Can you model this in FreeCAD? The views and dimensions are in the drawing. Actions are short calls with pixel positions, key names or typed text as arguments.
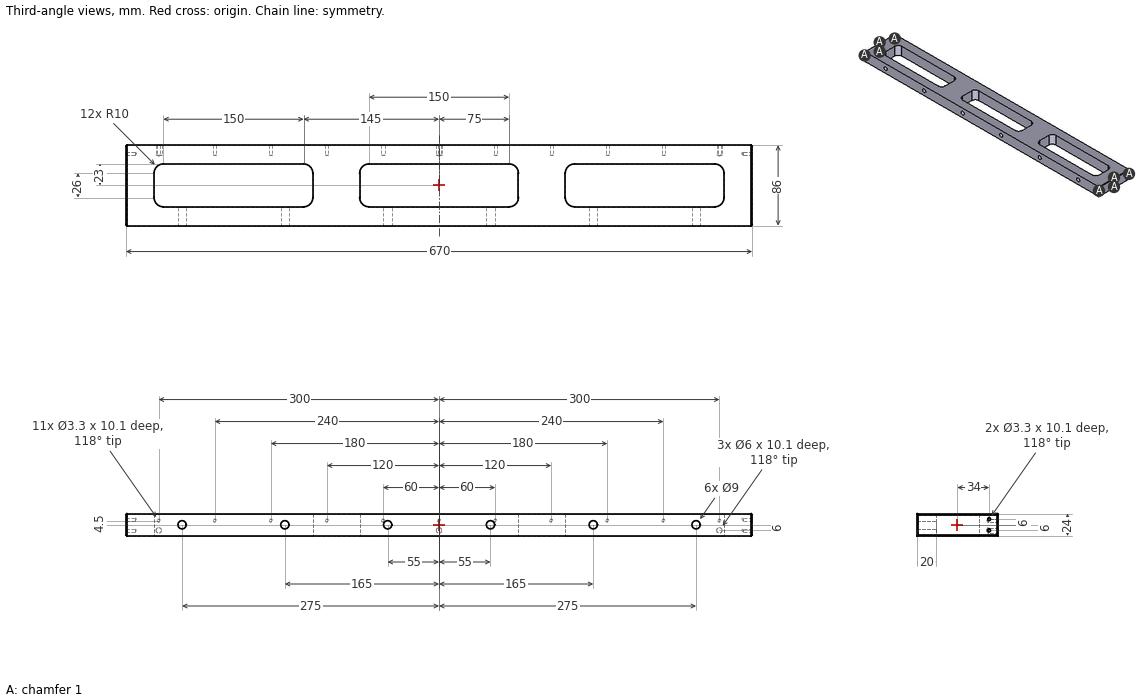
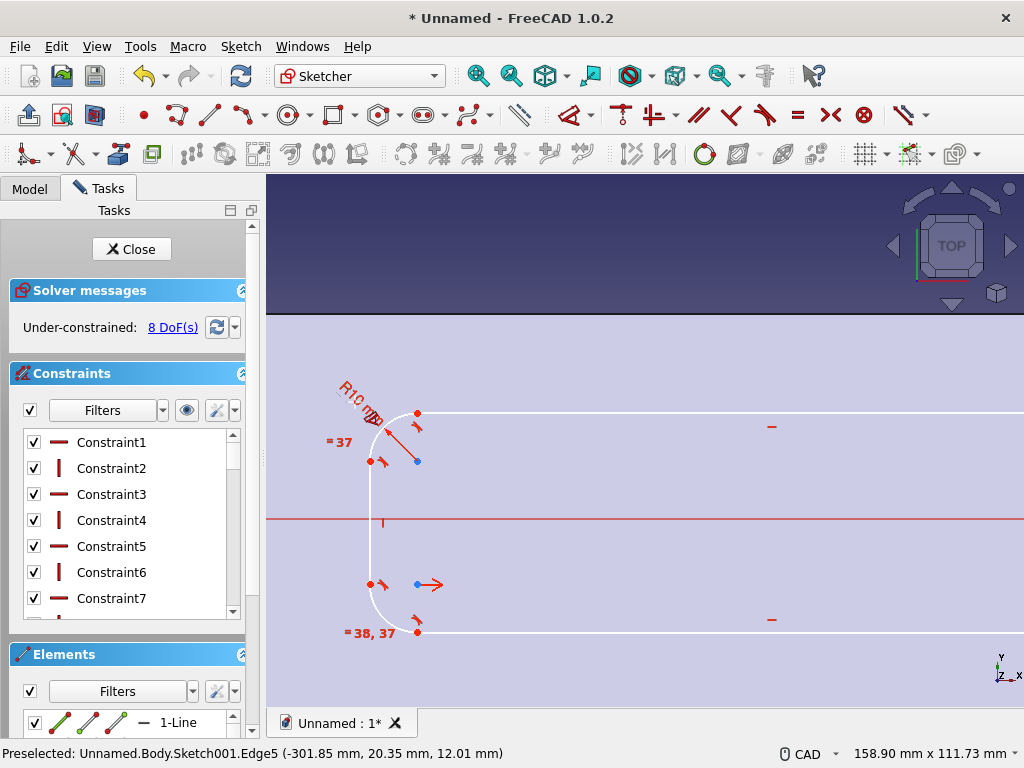
click(370, 498)
click(336, 495)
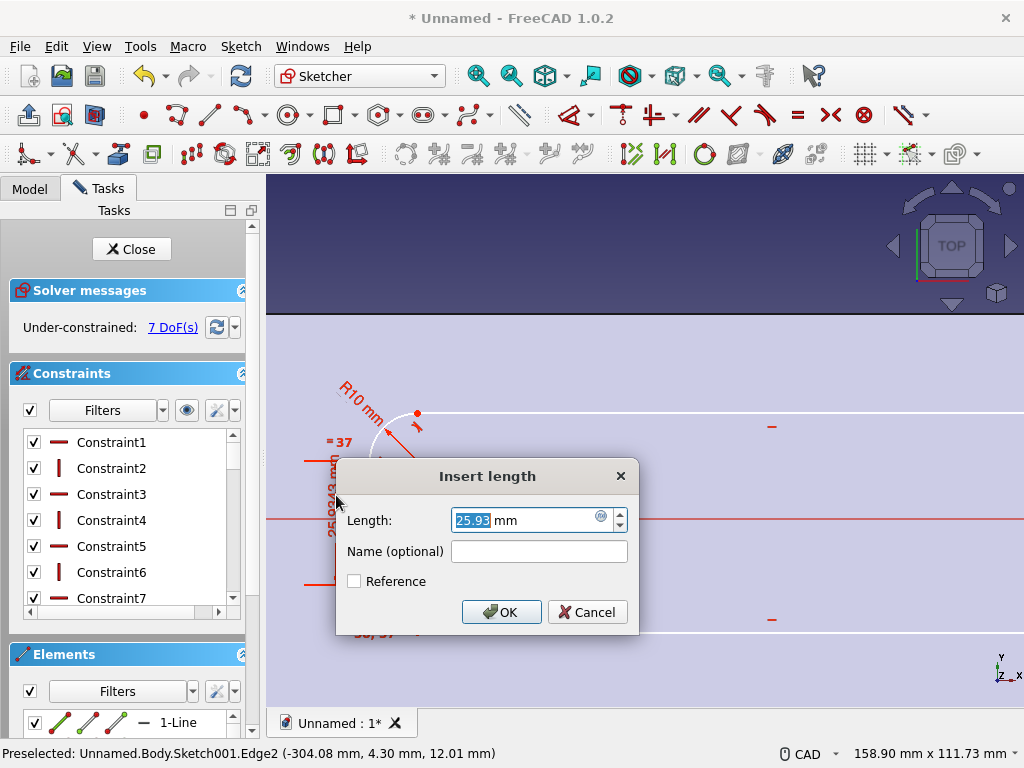
text(26)
key(Return)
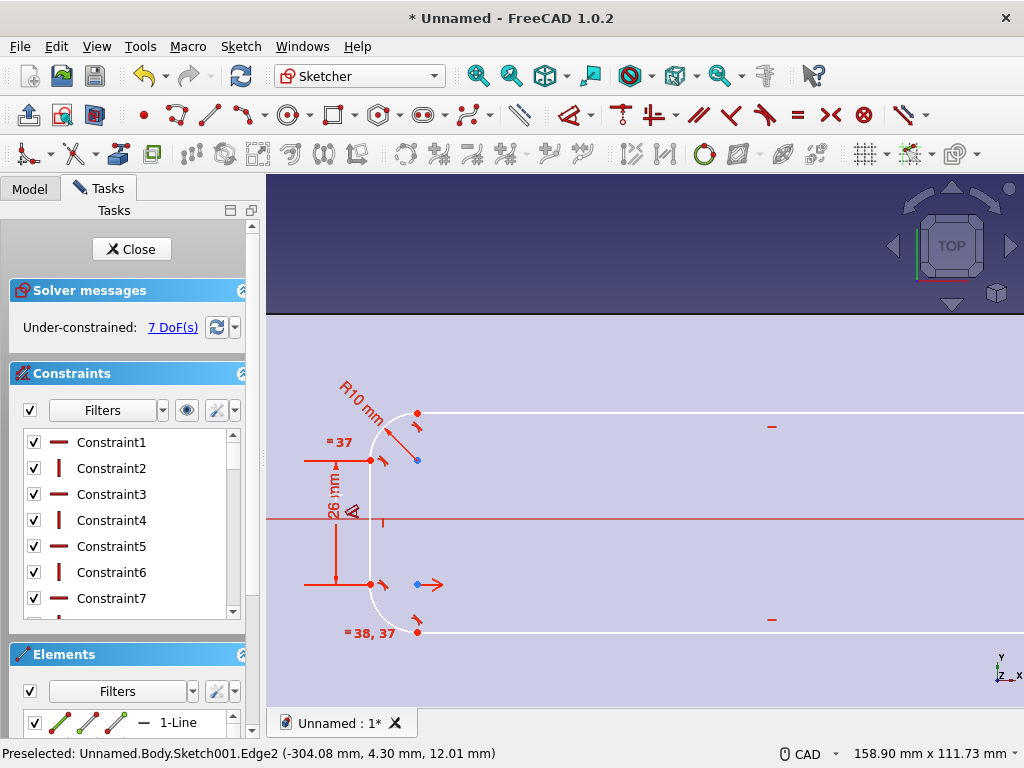
scroll(382, 428, down, 10)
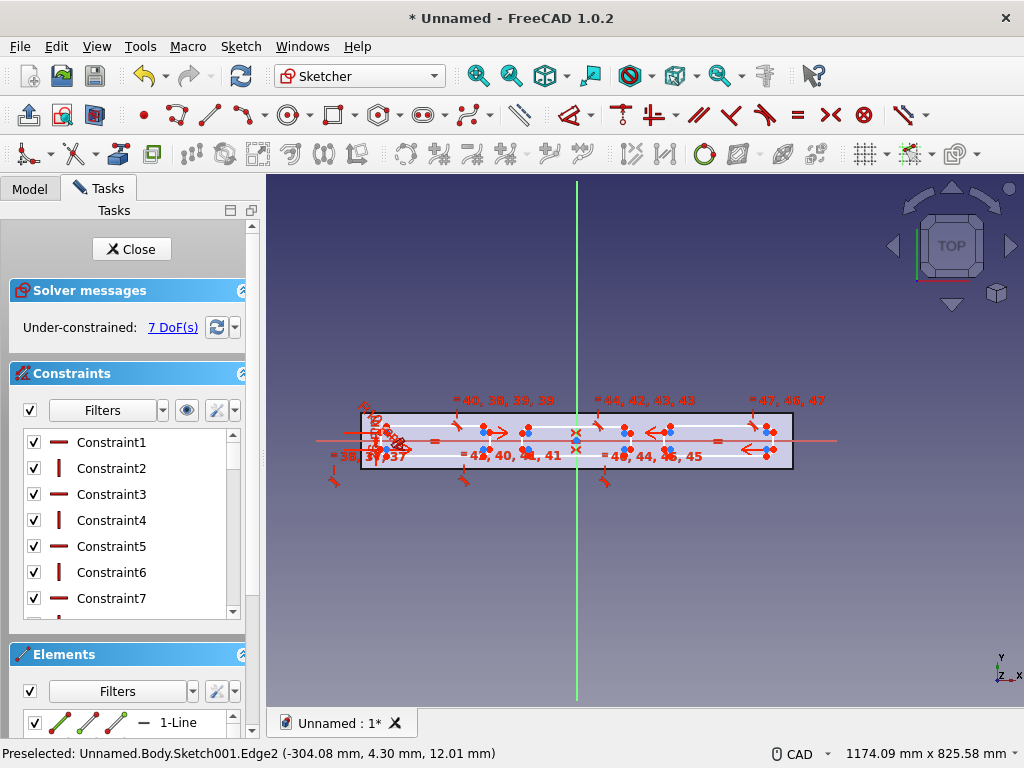
scroll(522, 438, up, 9)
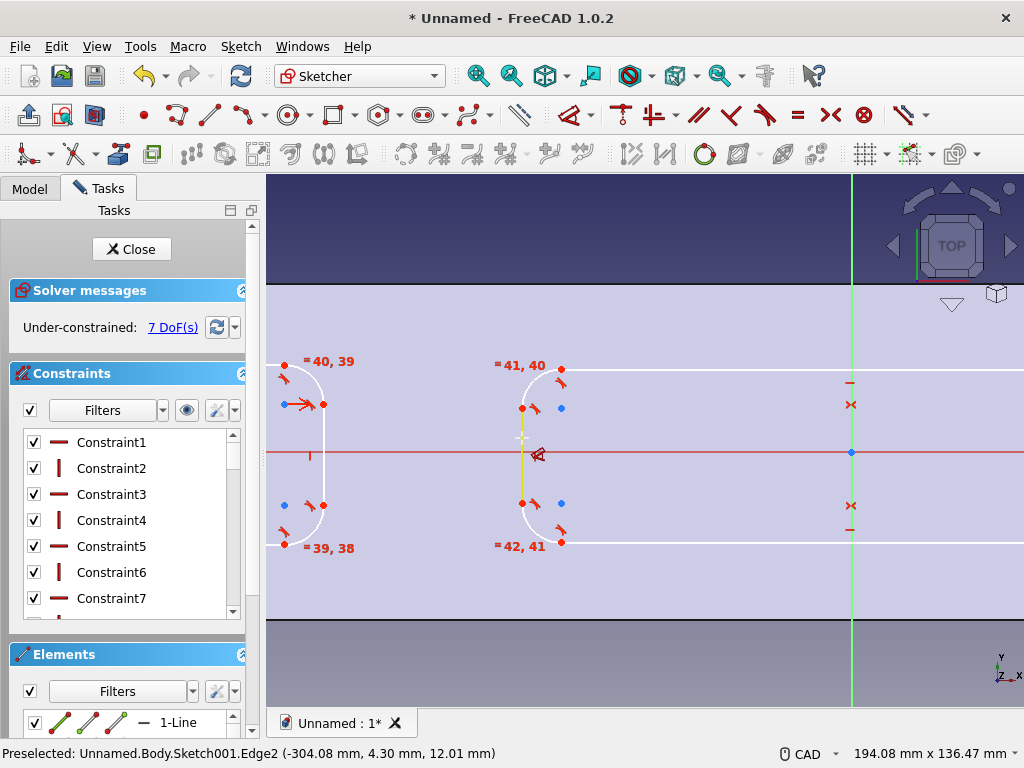
click(522, 437)
click(488, 434)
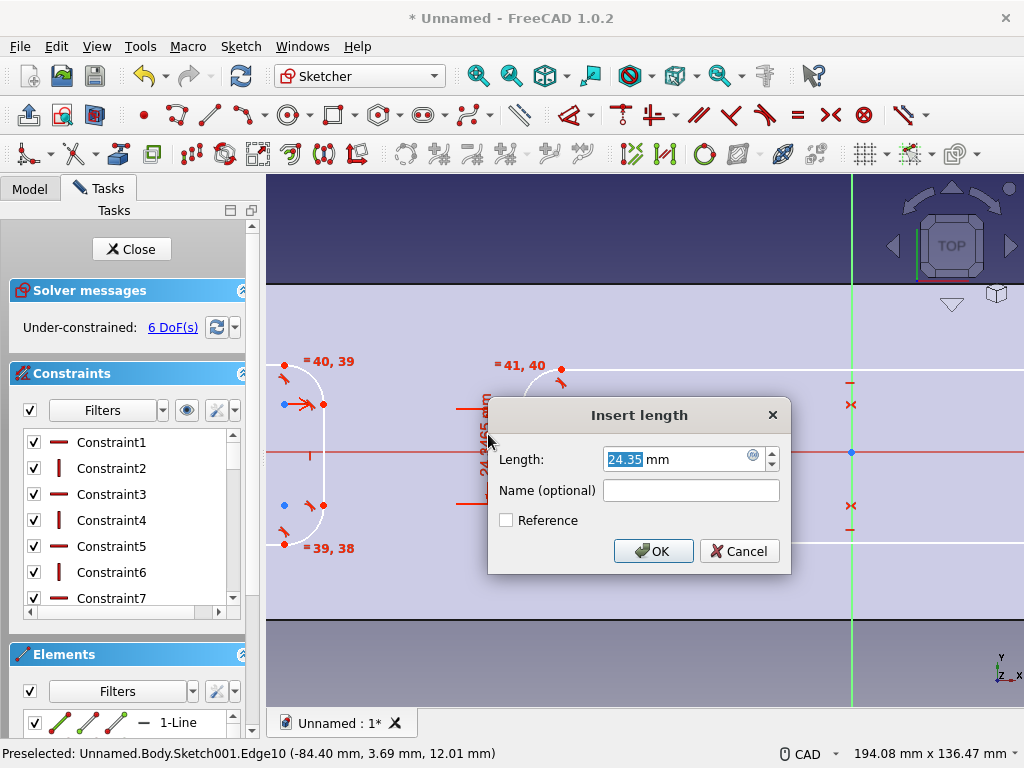
text(26)
key(Return)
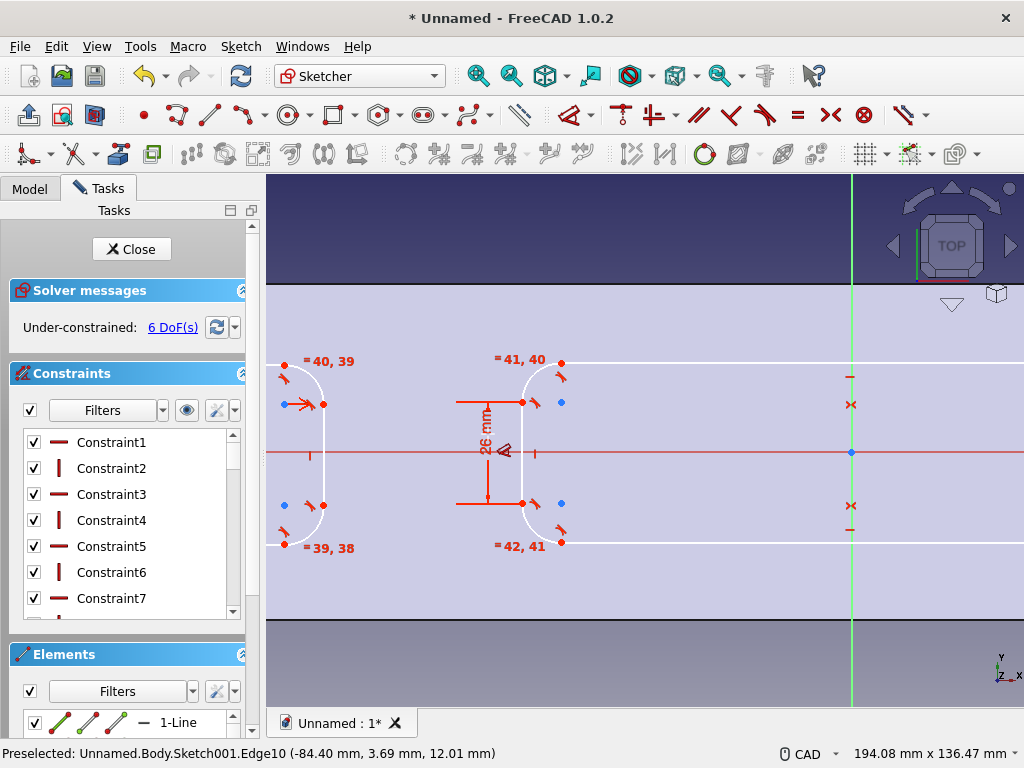
scroll(522, 438, down, 9)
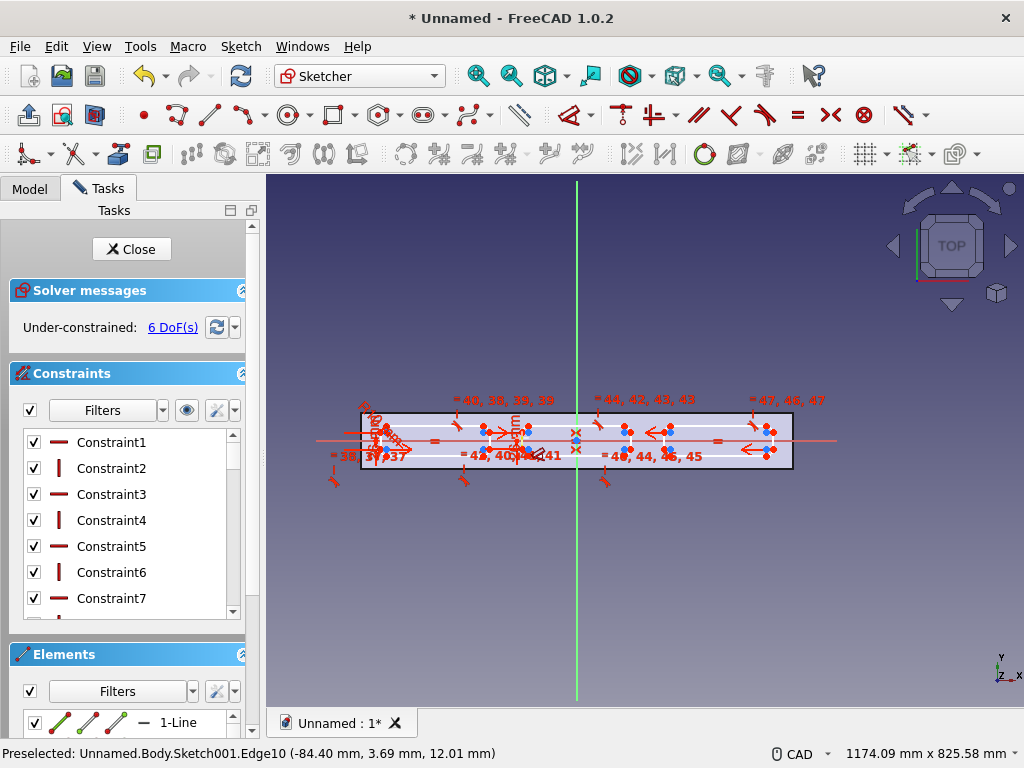
click(454, 426)
click(435, 392)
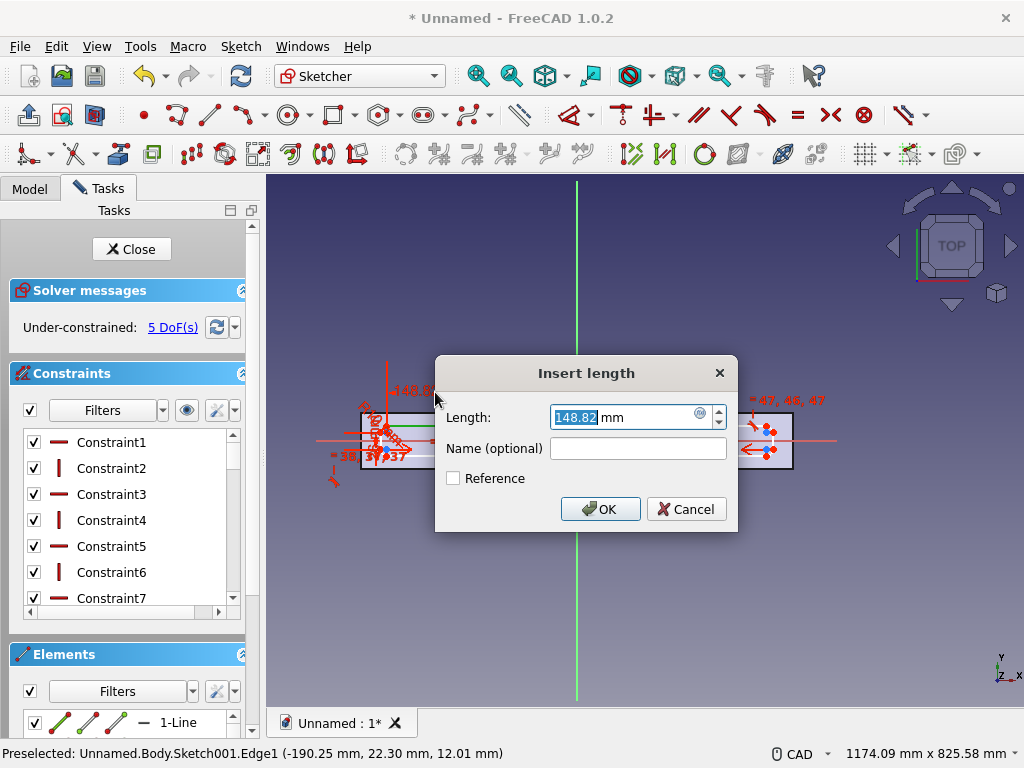
text(150)
key(Return)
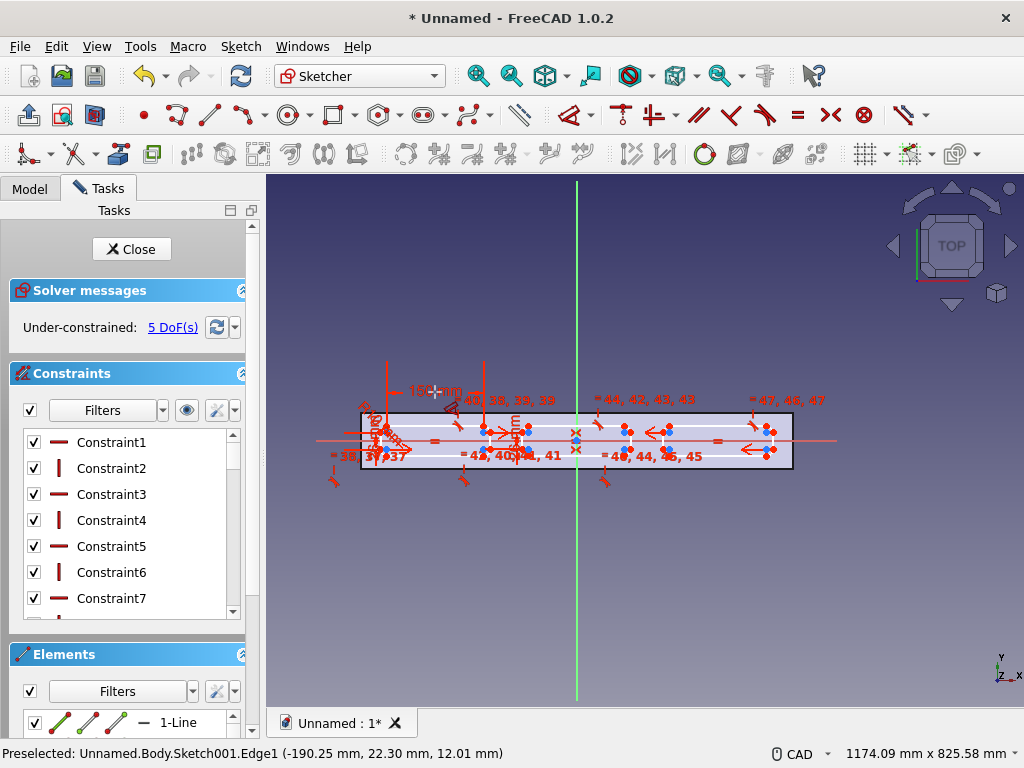
click(596, 426)
click(555, 392)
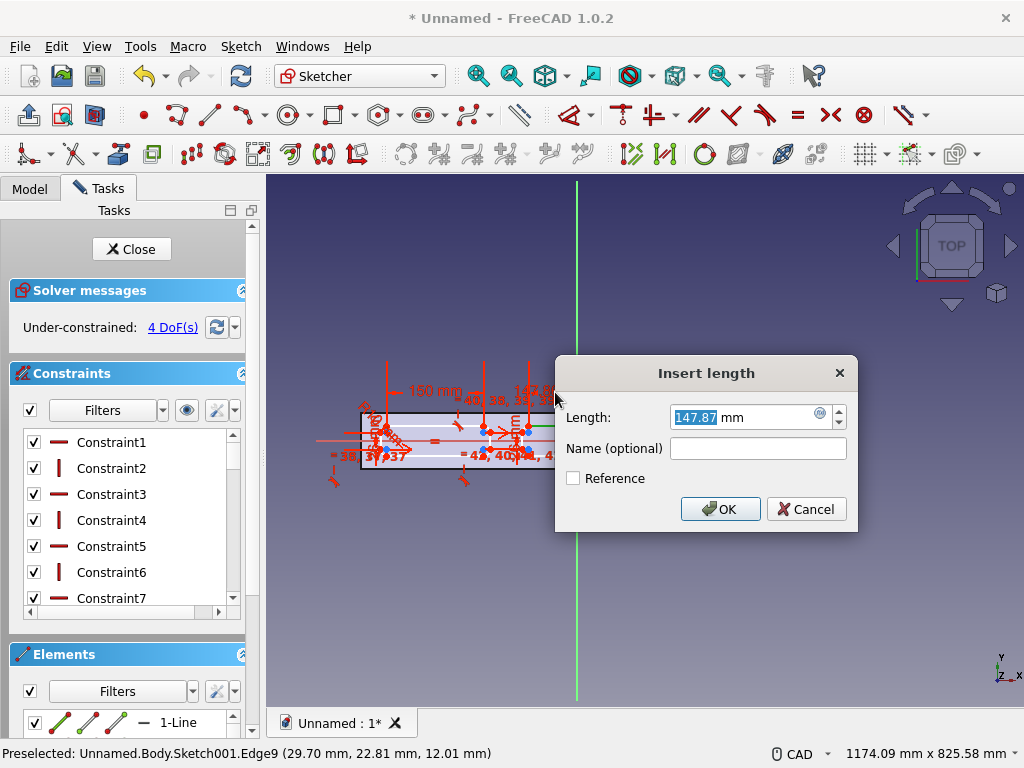
text(150)
key(Return)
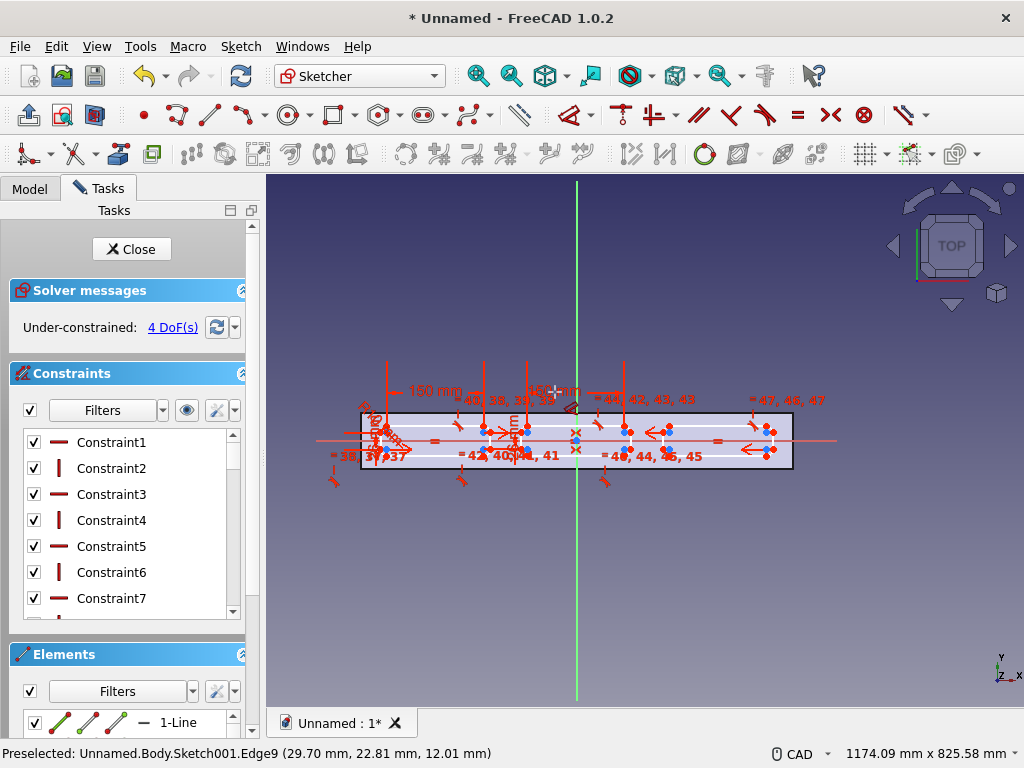
scroll(484, 426, up, 5)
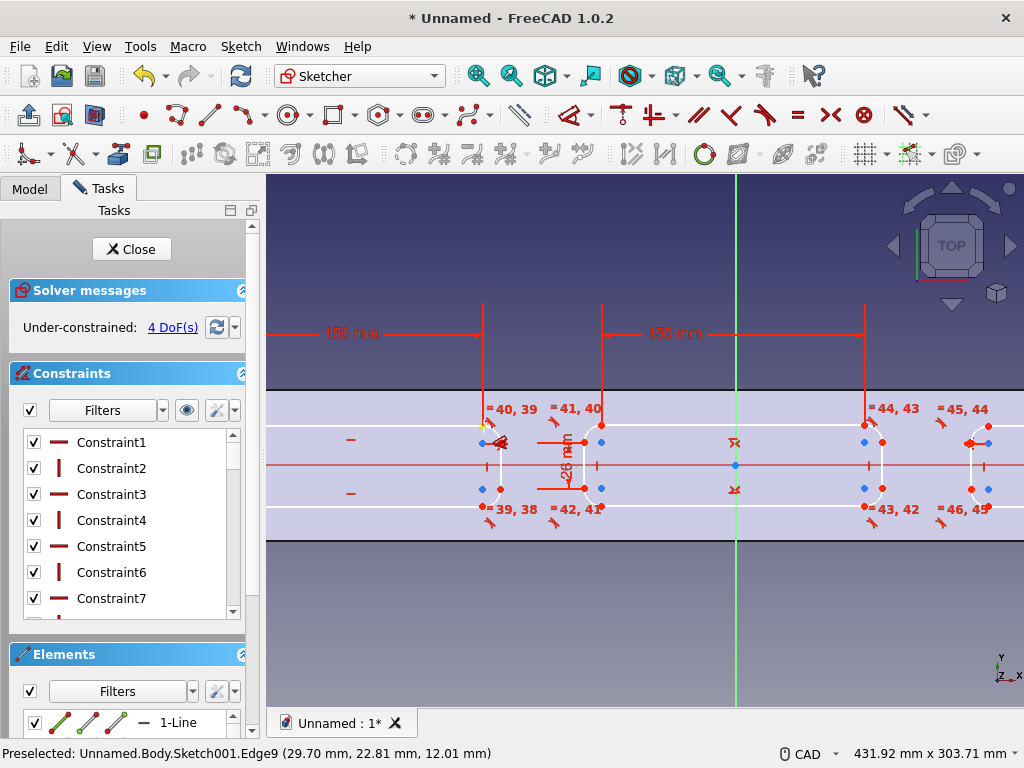
click(483, 426)
click(449, 446)